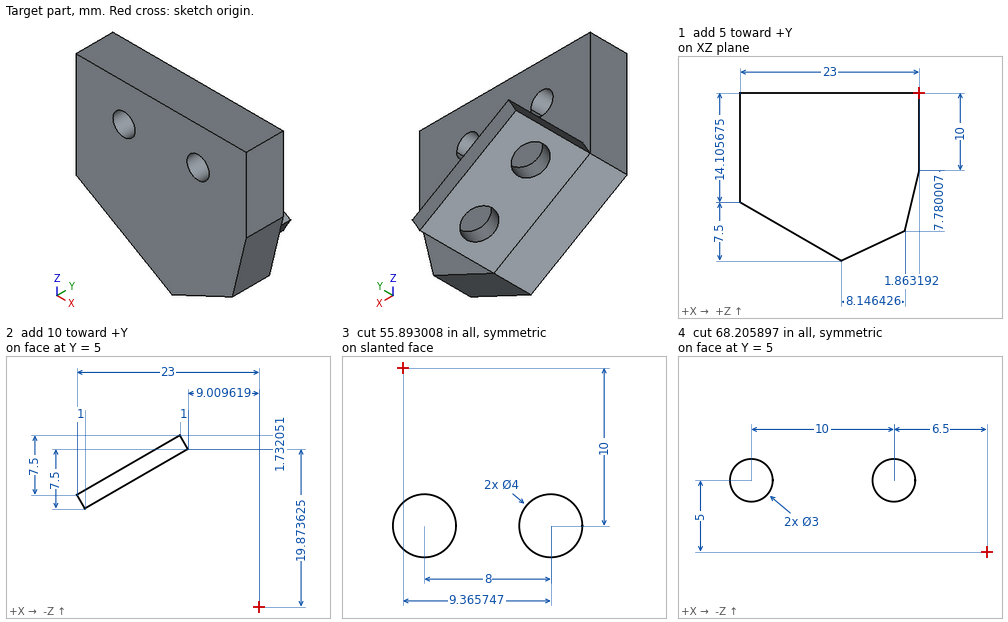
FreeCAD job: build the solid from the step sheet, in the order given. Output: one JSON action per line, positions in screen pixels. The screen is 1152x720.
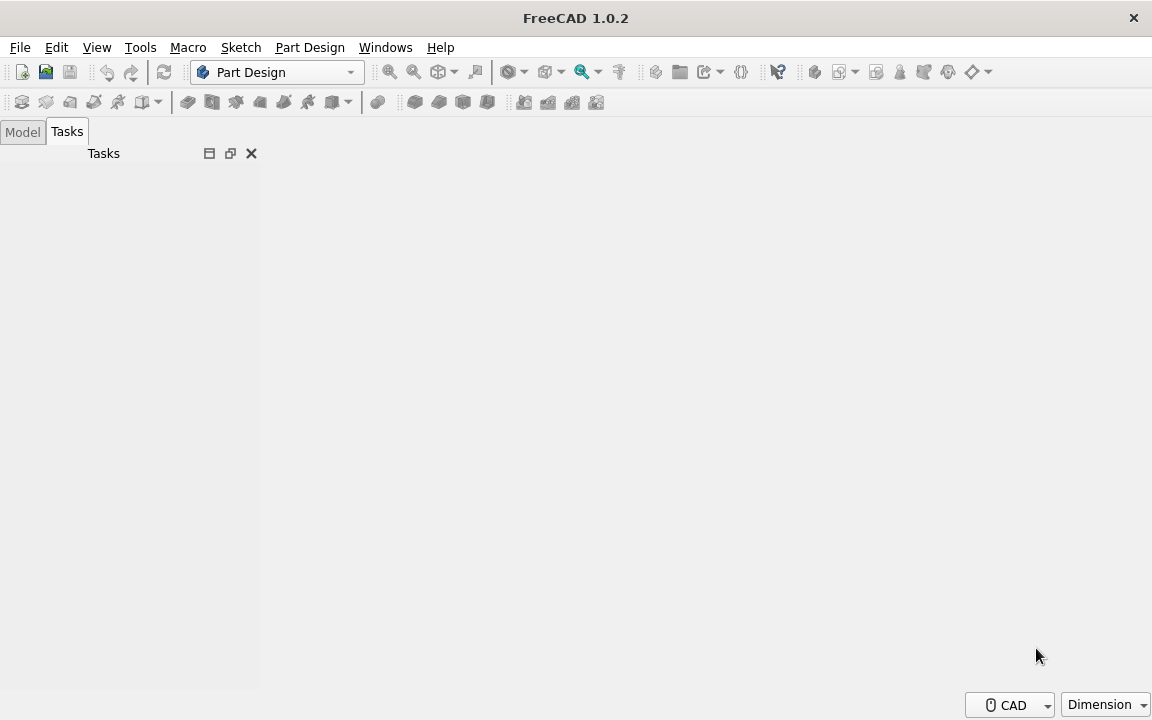
{"action": "left_click", "coordinate": [22, 72]}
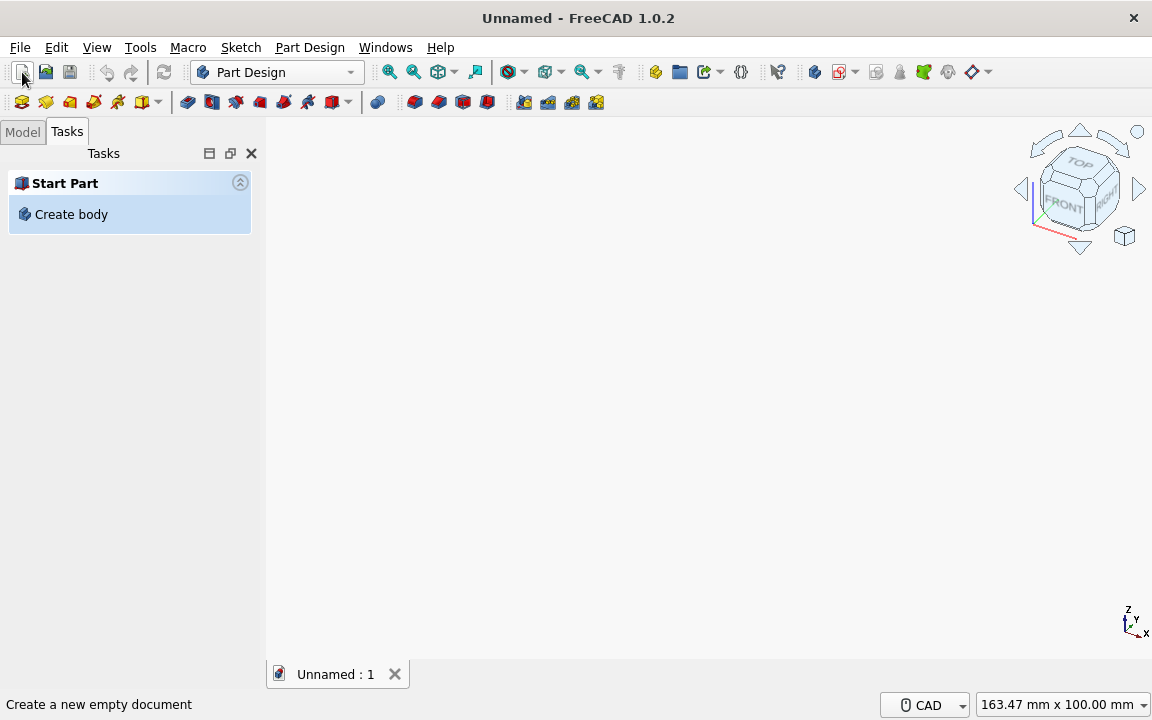
{"action": "left_click", "coordinate": [840, 72]}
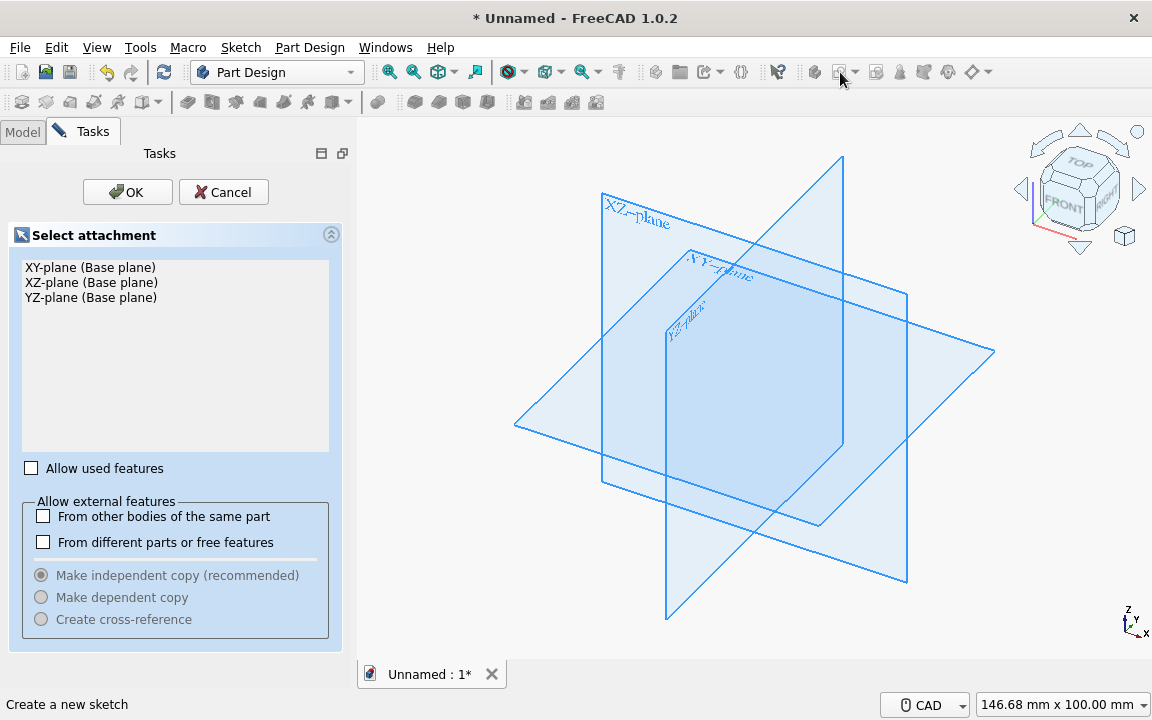
{"action": "left_click", "coordinate": [82, 282]}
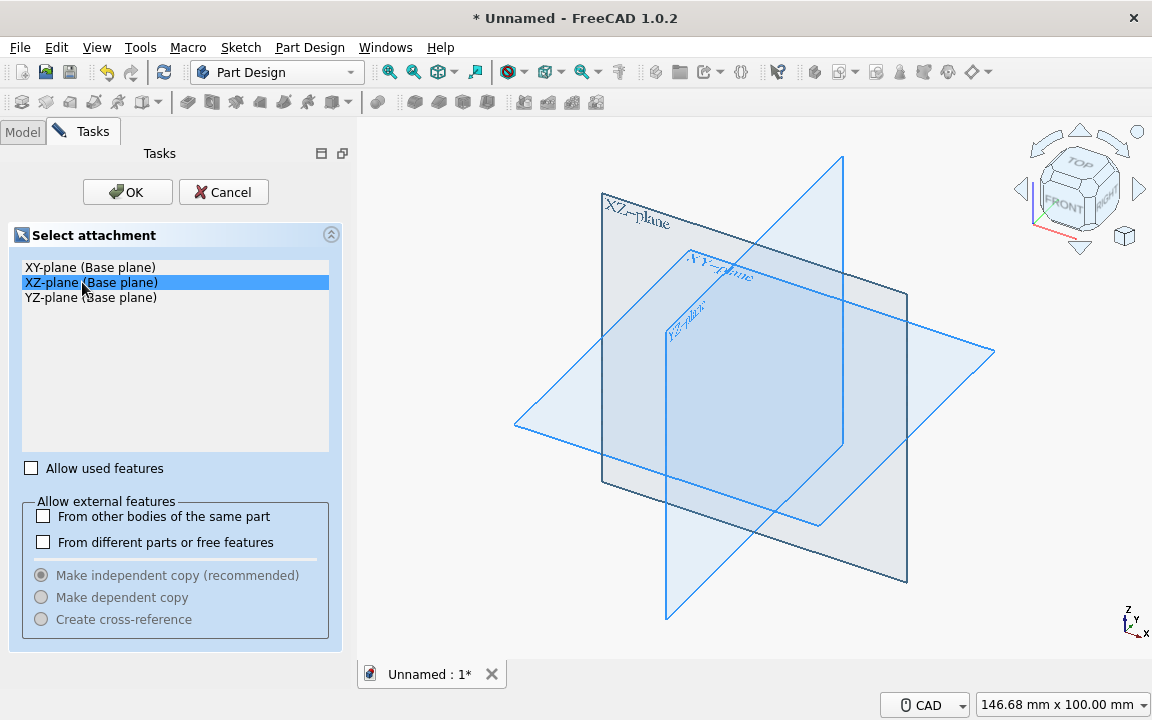
{"action": "left_click", "coordinate": [128, 192]}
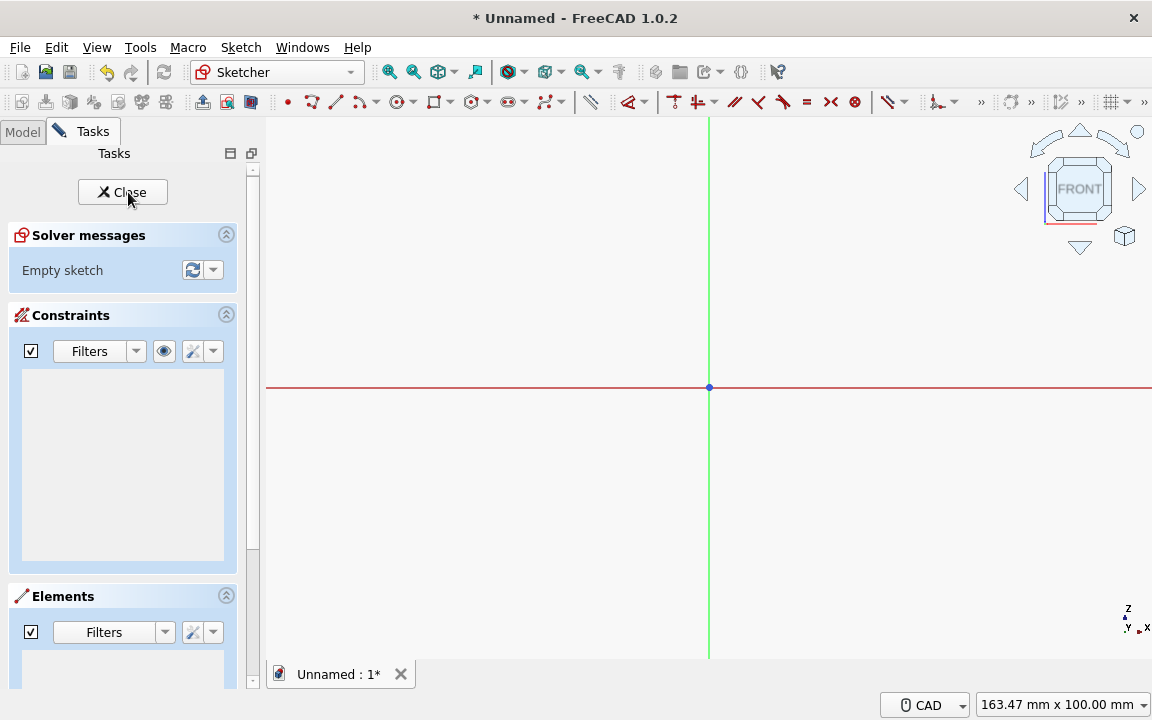
{"action": "scroll", "coordinate": [650, 481], "scroll_direction": "up", "scroll_amount": 5}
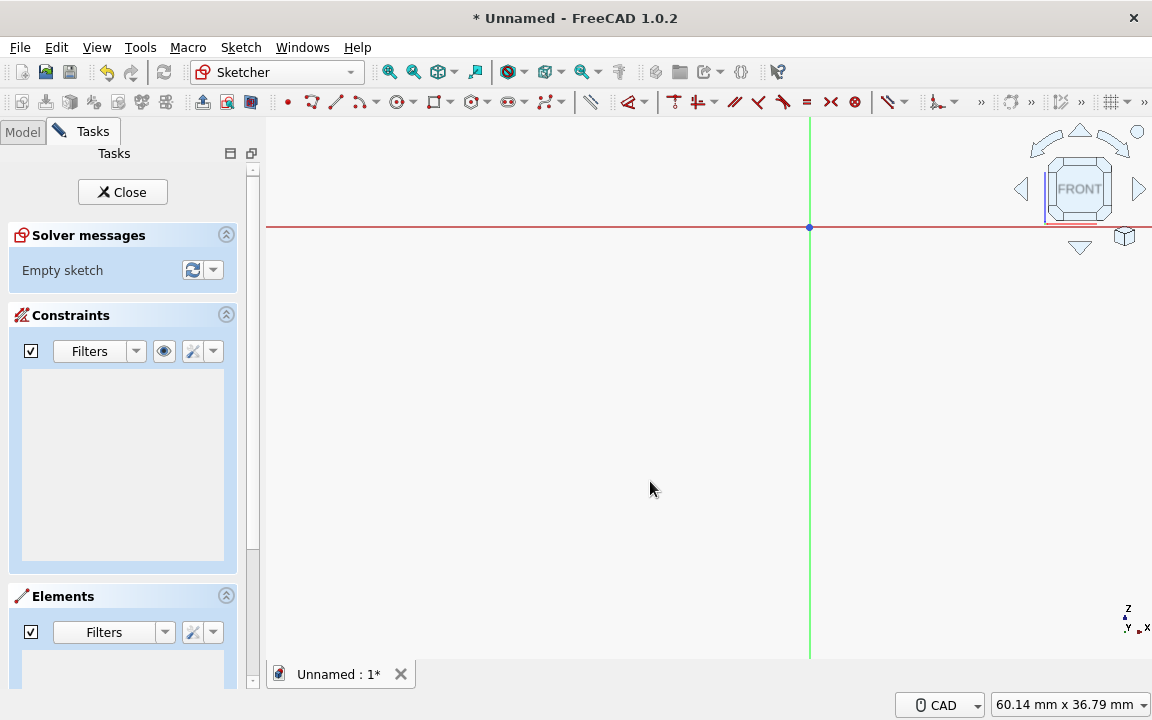
{"action": "left_click", "coordinate": [312, 102]}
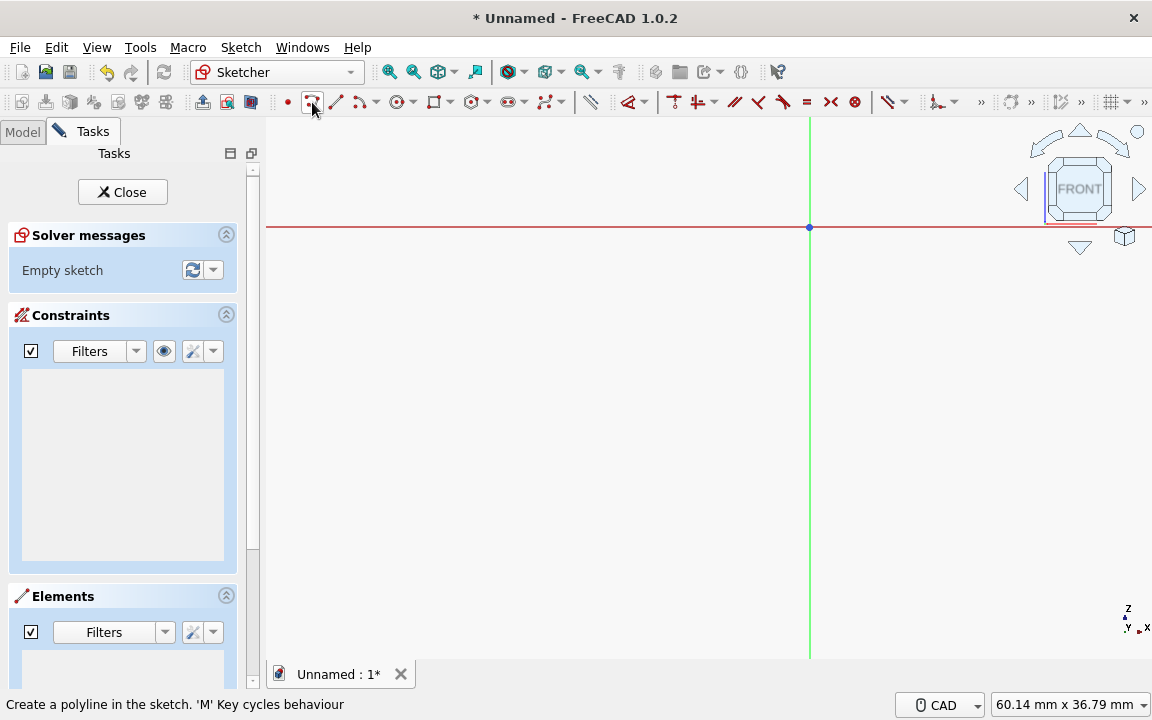
{"action": "left_click", "coordinate": [810, 227]}
{"action": "left_click", "coordinate": [801, 374]}
{"action": "left_click", "coordinate": [782, 489]}
{"action": "left_click", "coordinate": [662, 545]}
{"action": "left_click", "coordinate": [471, 435]}
{"action": "left_click", "coordinate": [471, 236]}
{"action": "left_click", "coordinate": [810, 227]}
{"action": "key", "text": "Escape"}
{"action": "key", "text": "Escape"}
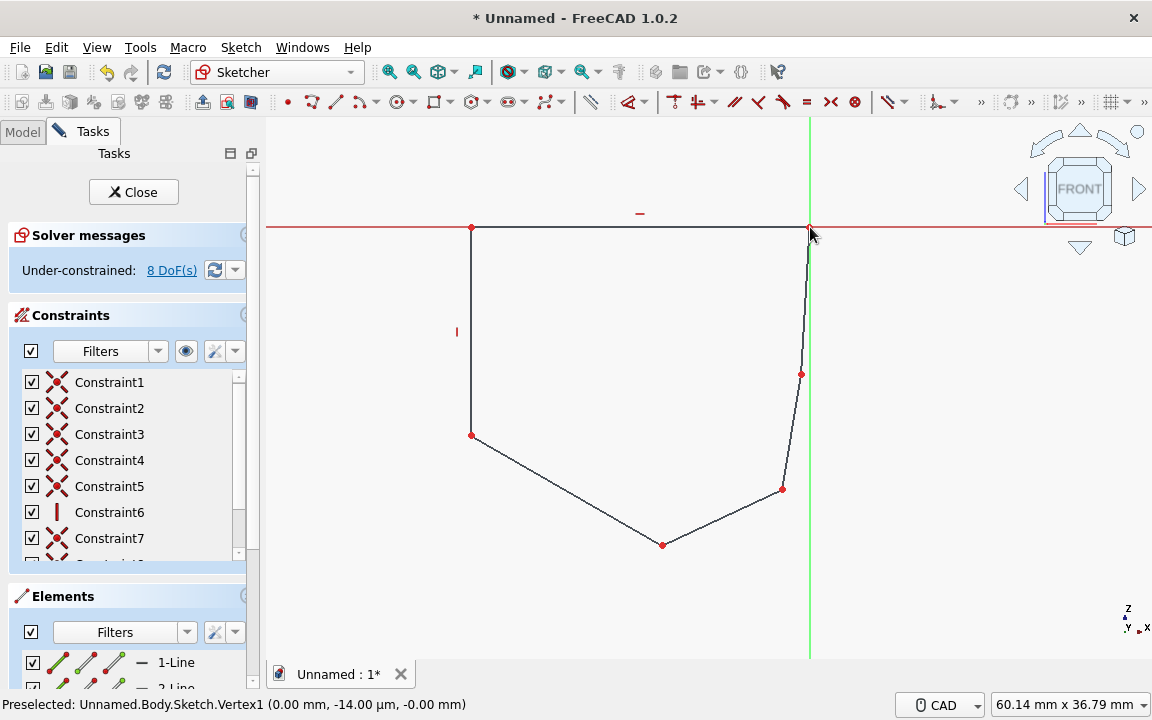
{"action": "left_click", "coordinate": [807, 271]}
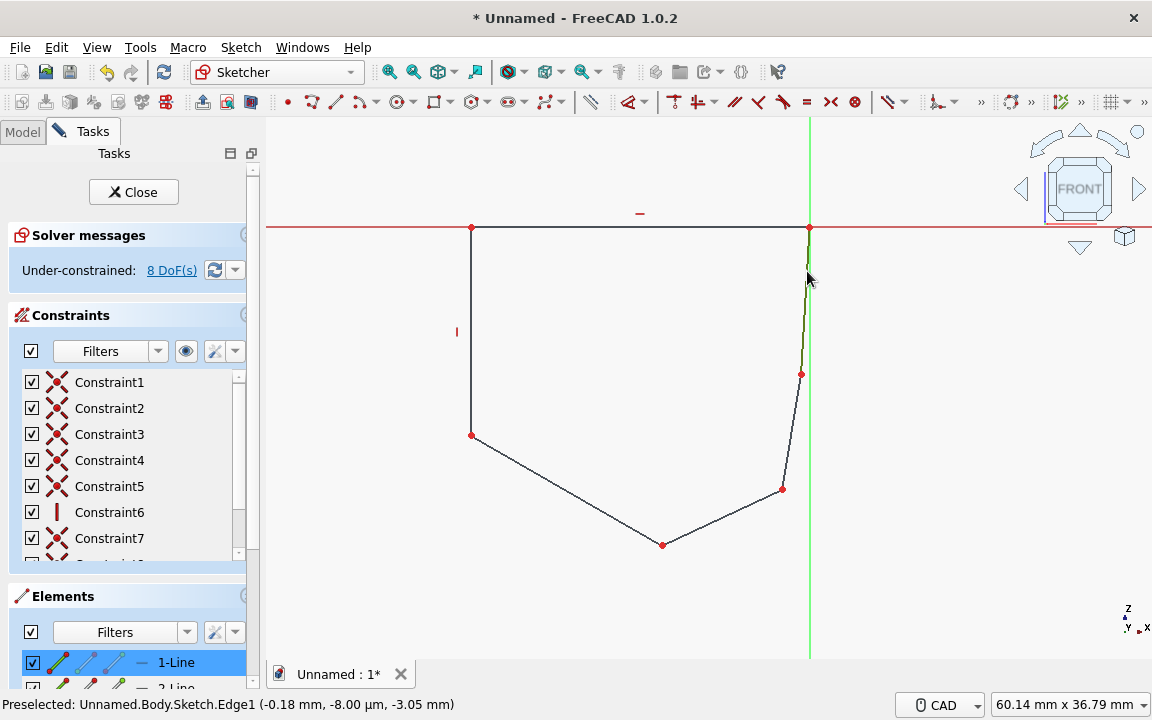
{"action": "left_click", "coordinate": [716, 102]}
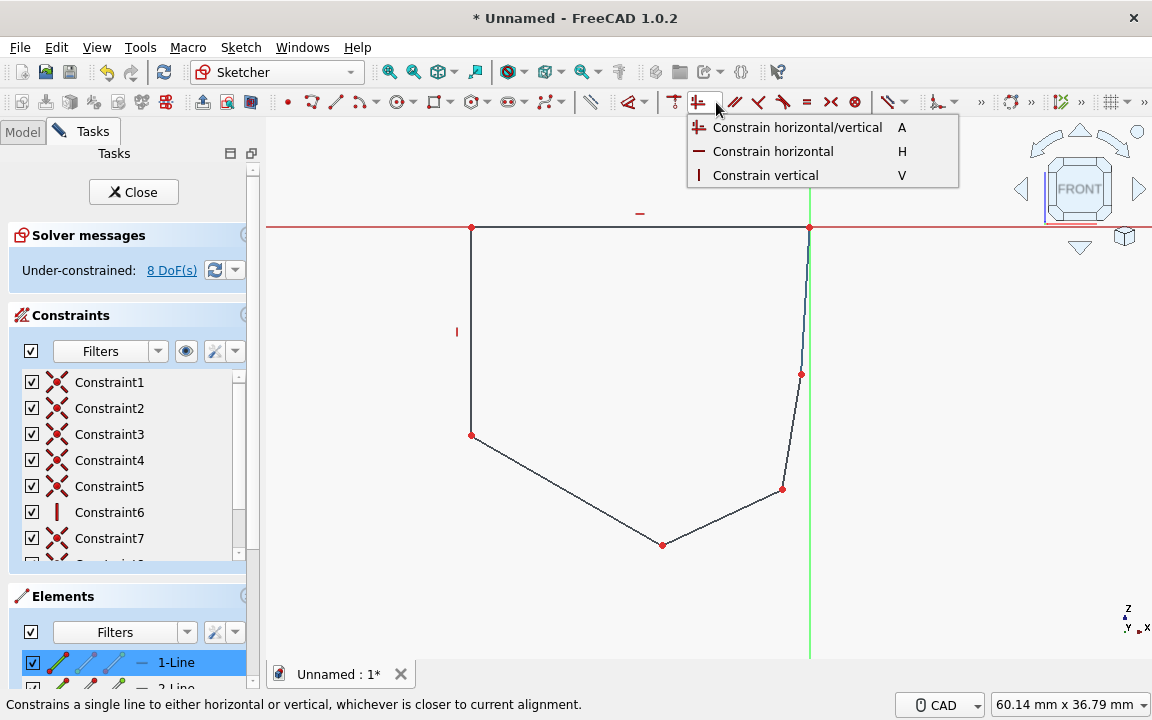
{"action": "left_click", "coordinate": [823, 175]}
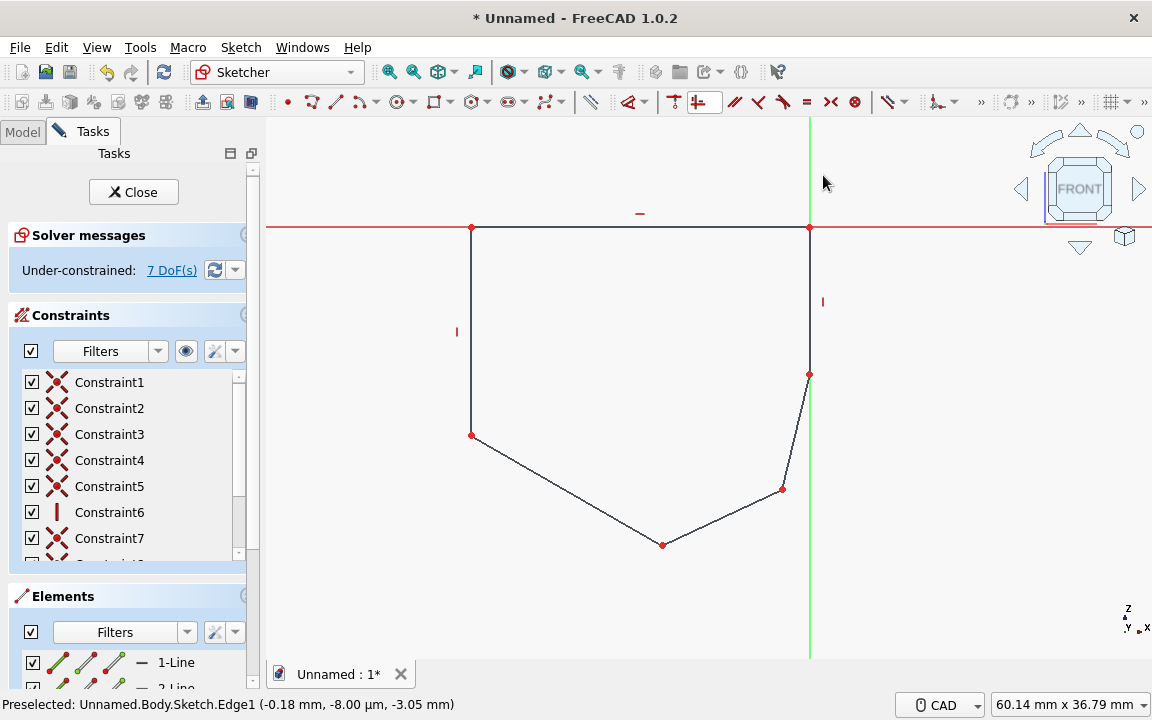
{"action": "left_click", "coordinate": [810, 271]}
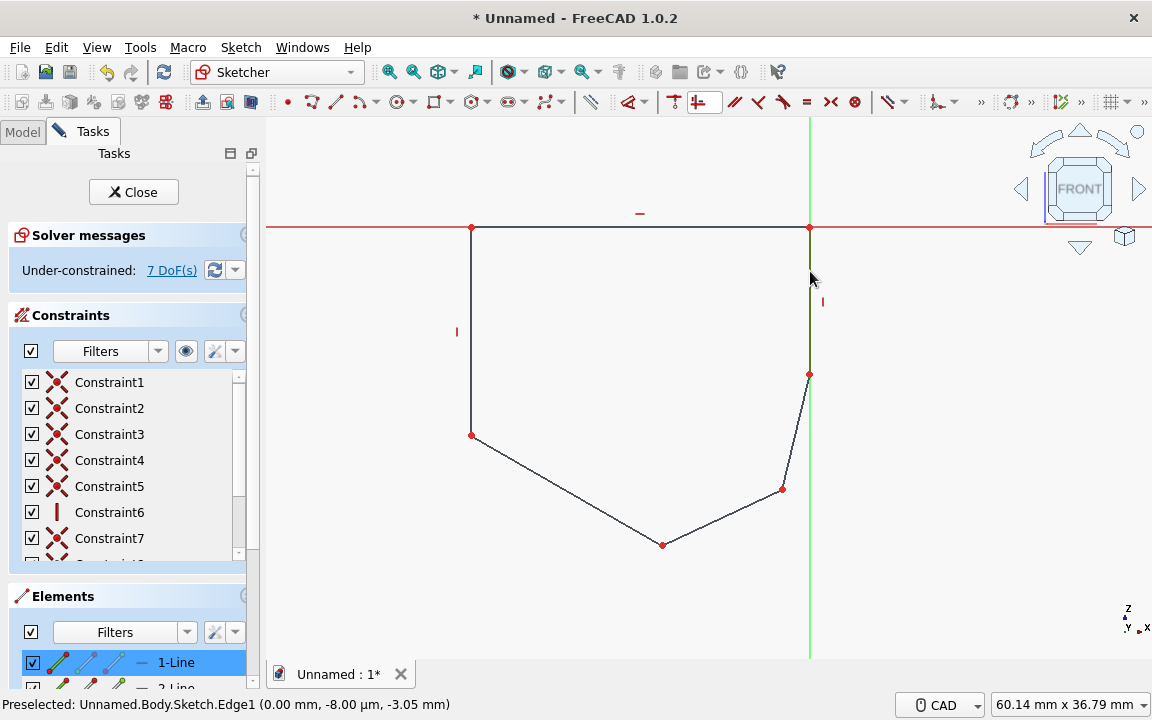
{"action": "left_click", "coordinate": [646, 102]}